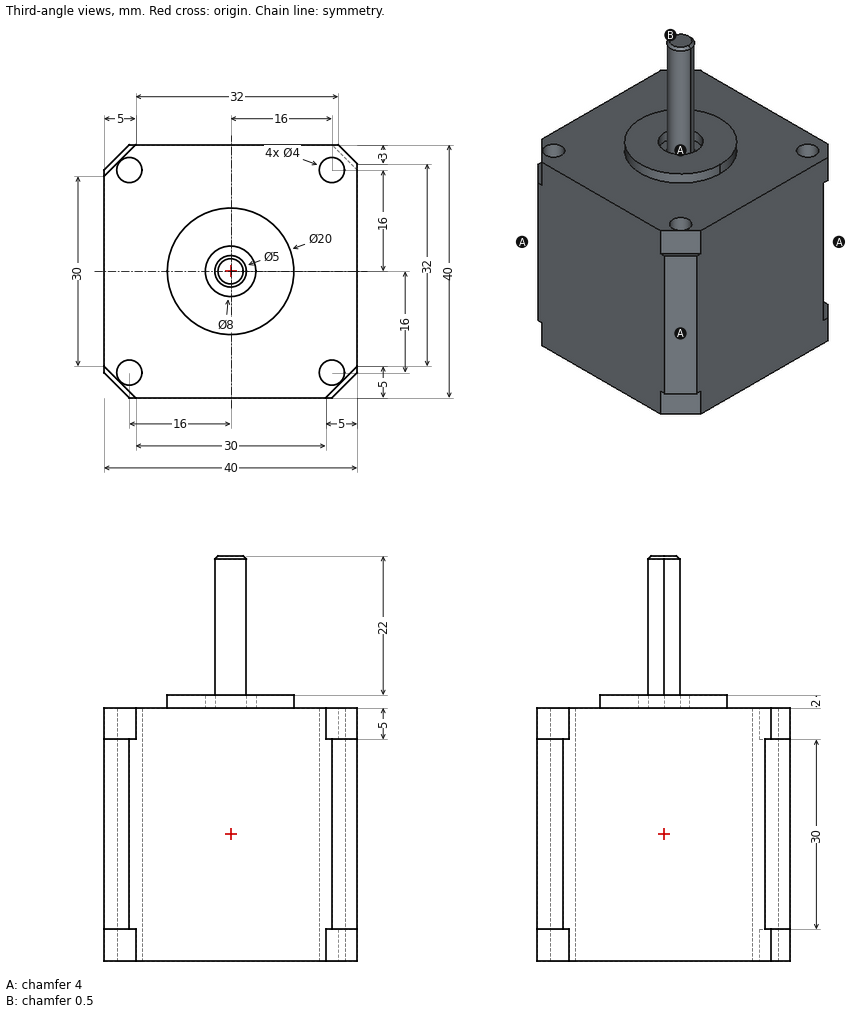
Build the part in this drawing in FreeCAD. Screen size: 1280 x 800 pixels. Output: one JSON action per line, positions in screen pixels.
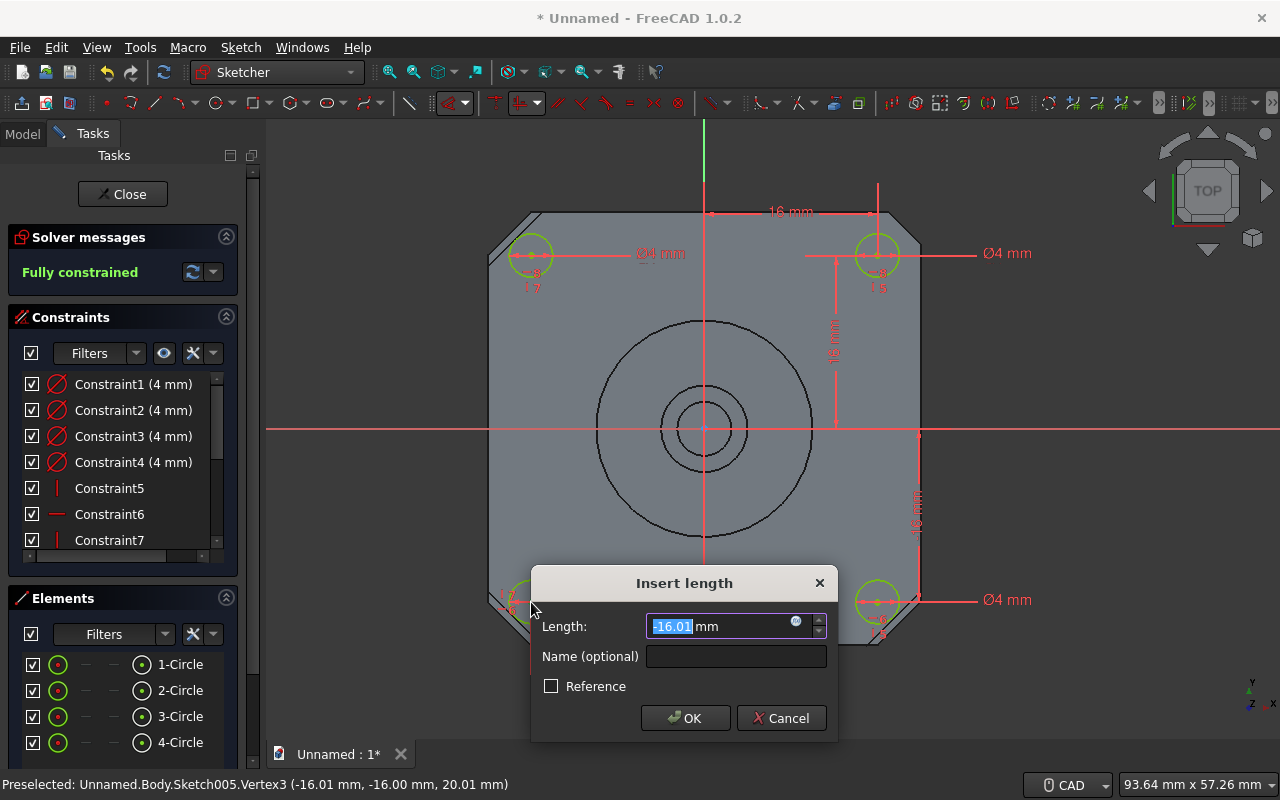
{"action": "type", "text": "-16"}
{"action": "key", "text": "Return"}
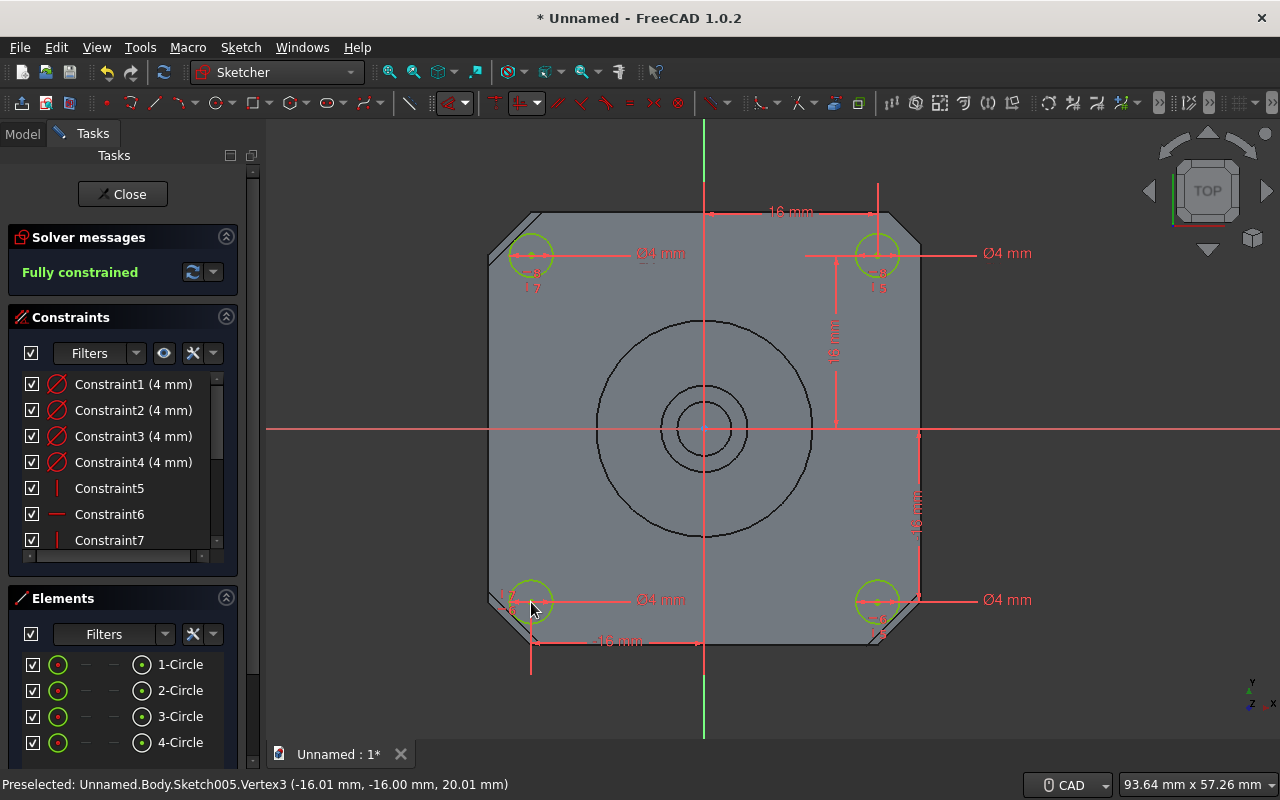
{"action": "left_click", "coordinate": [123, 194]}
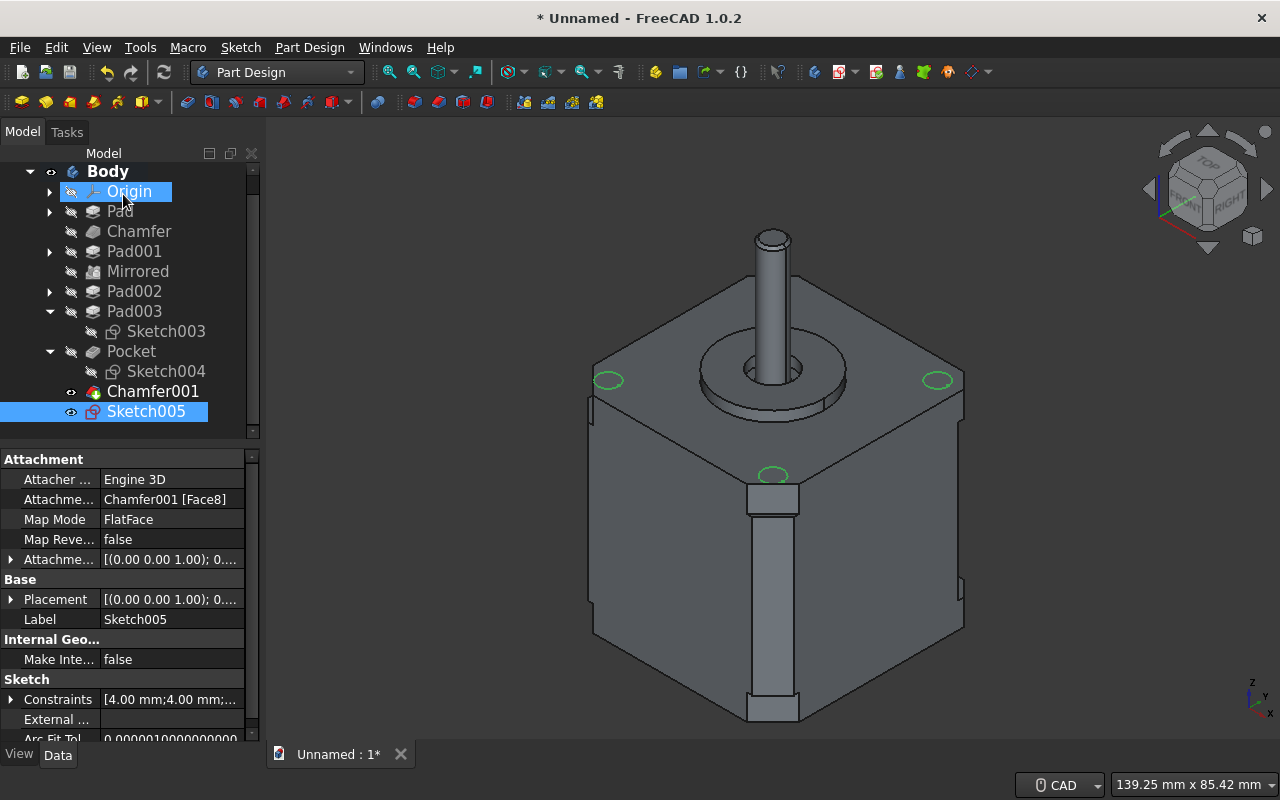
{"action": "left_click", "coordinate": [188, 102]}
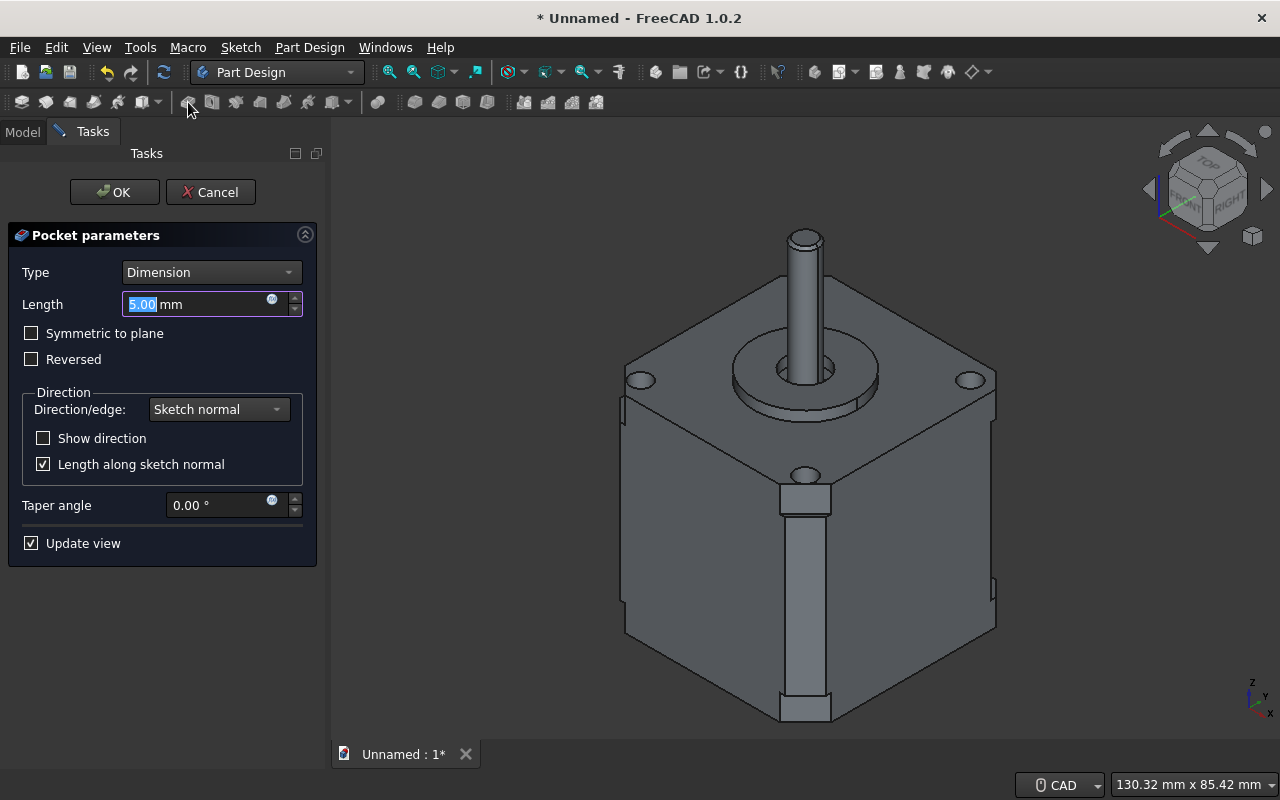
{"action": "left_click", "coordinate": [212, 272]}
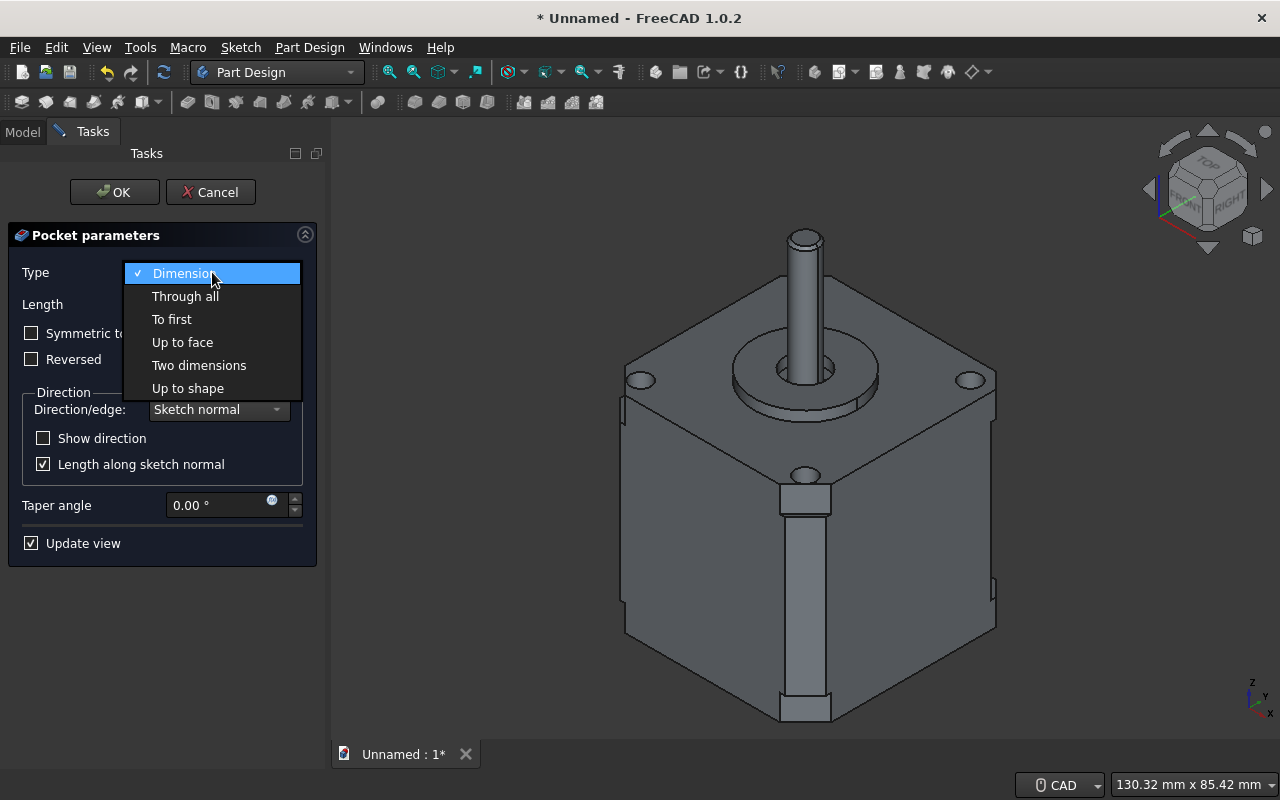
{"action": "left_click", "coordinate": [212, 296]}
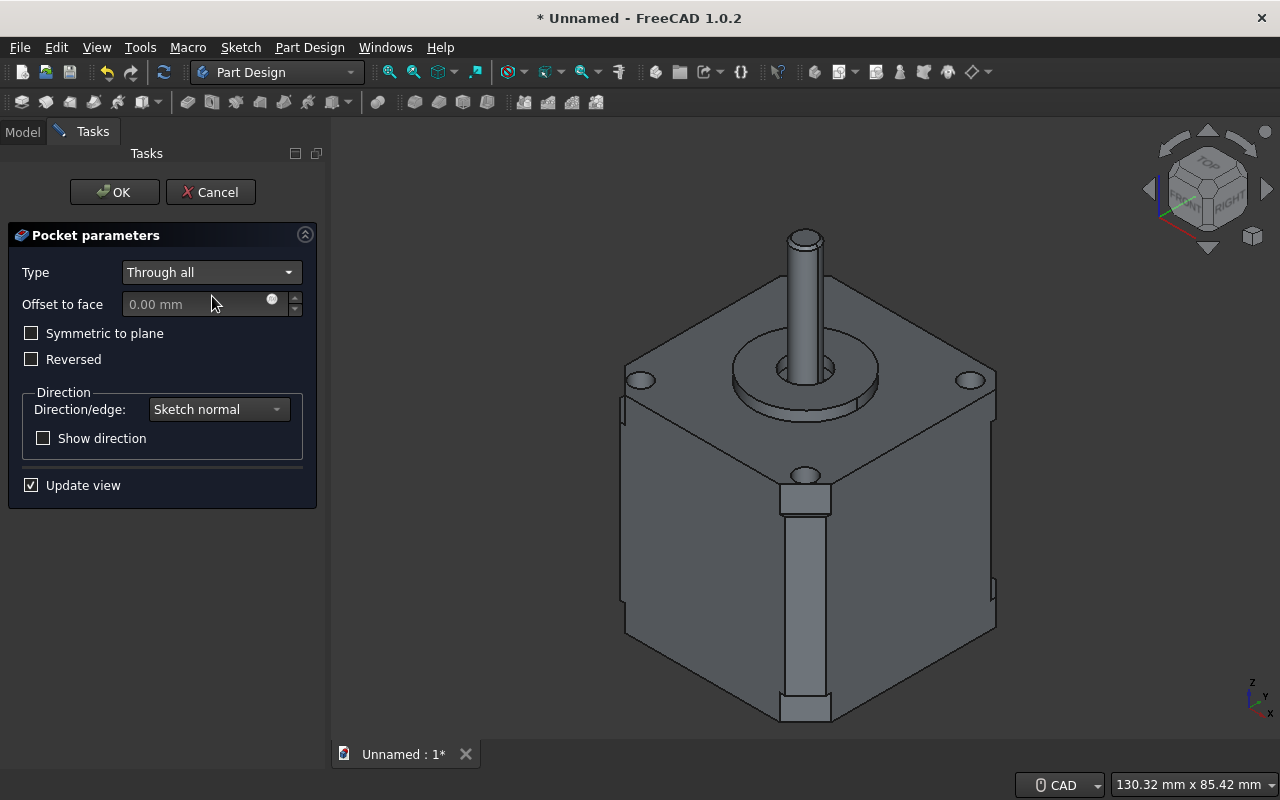
{"action": "left_click", "coordinate": [115, 192]}